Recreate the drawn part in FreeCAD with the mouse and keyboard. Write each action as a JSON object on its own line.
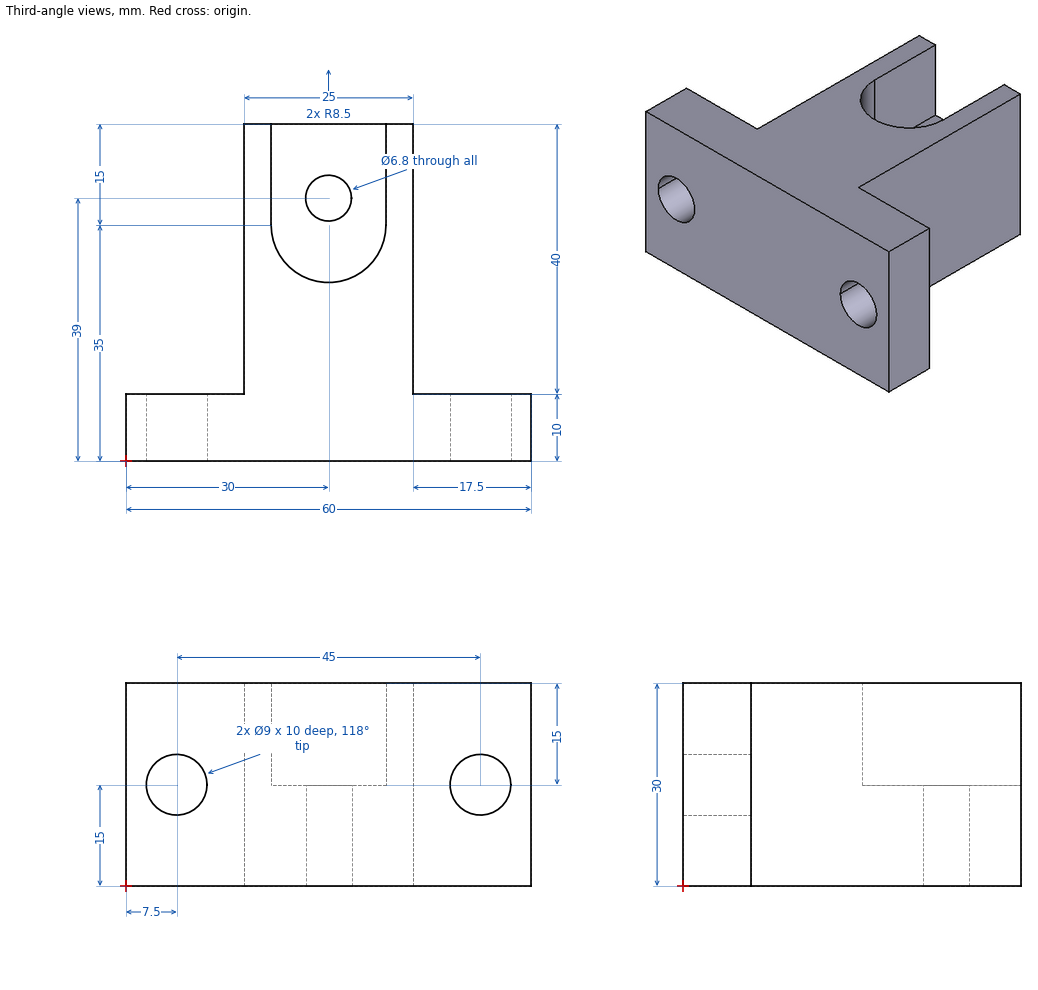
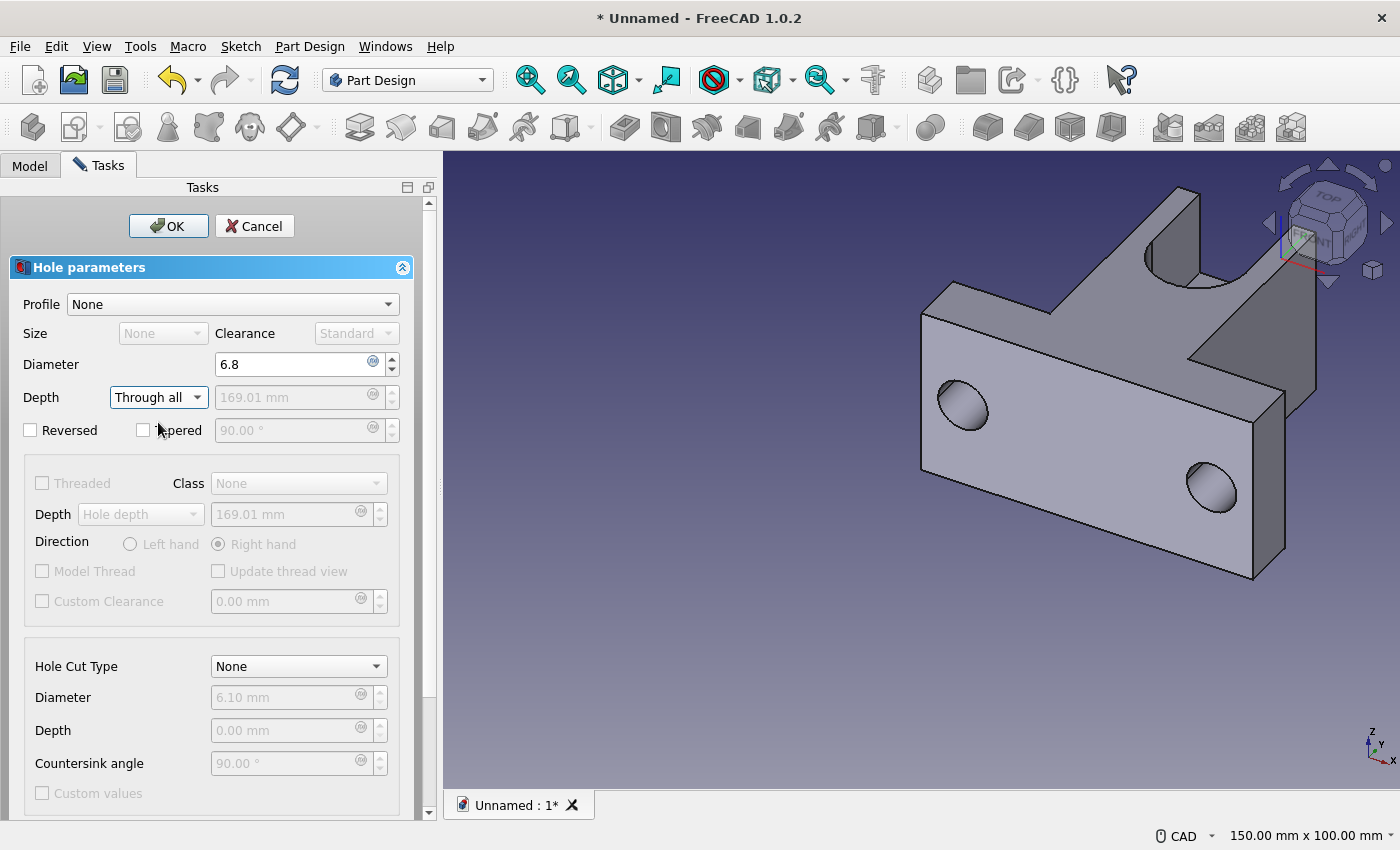
{"action": "left_click", "coordinate": [31, 430]}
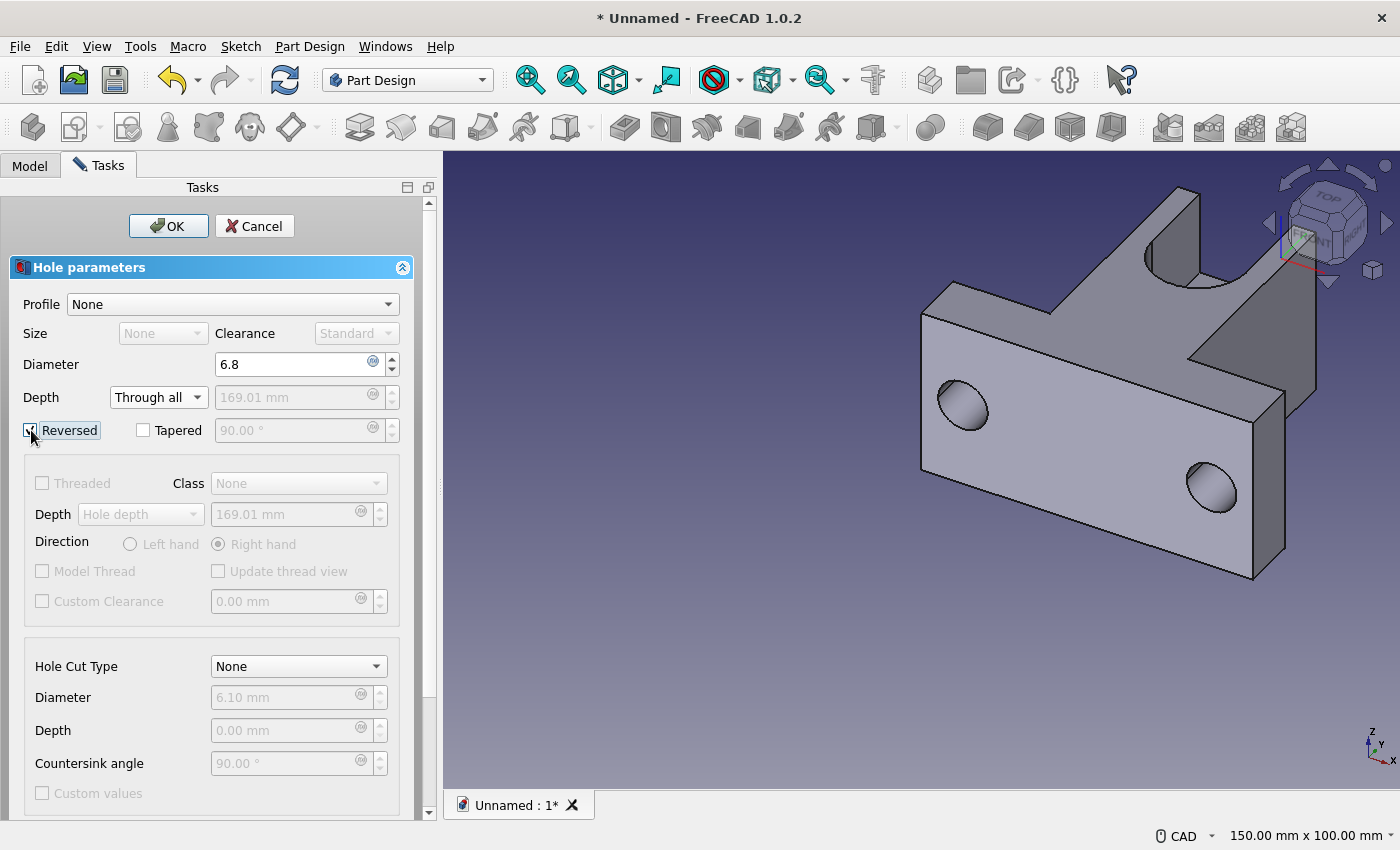
{"action": "left_click", "coordinate": [169, 226]}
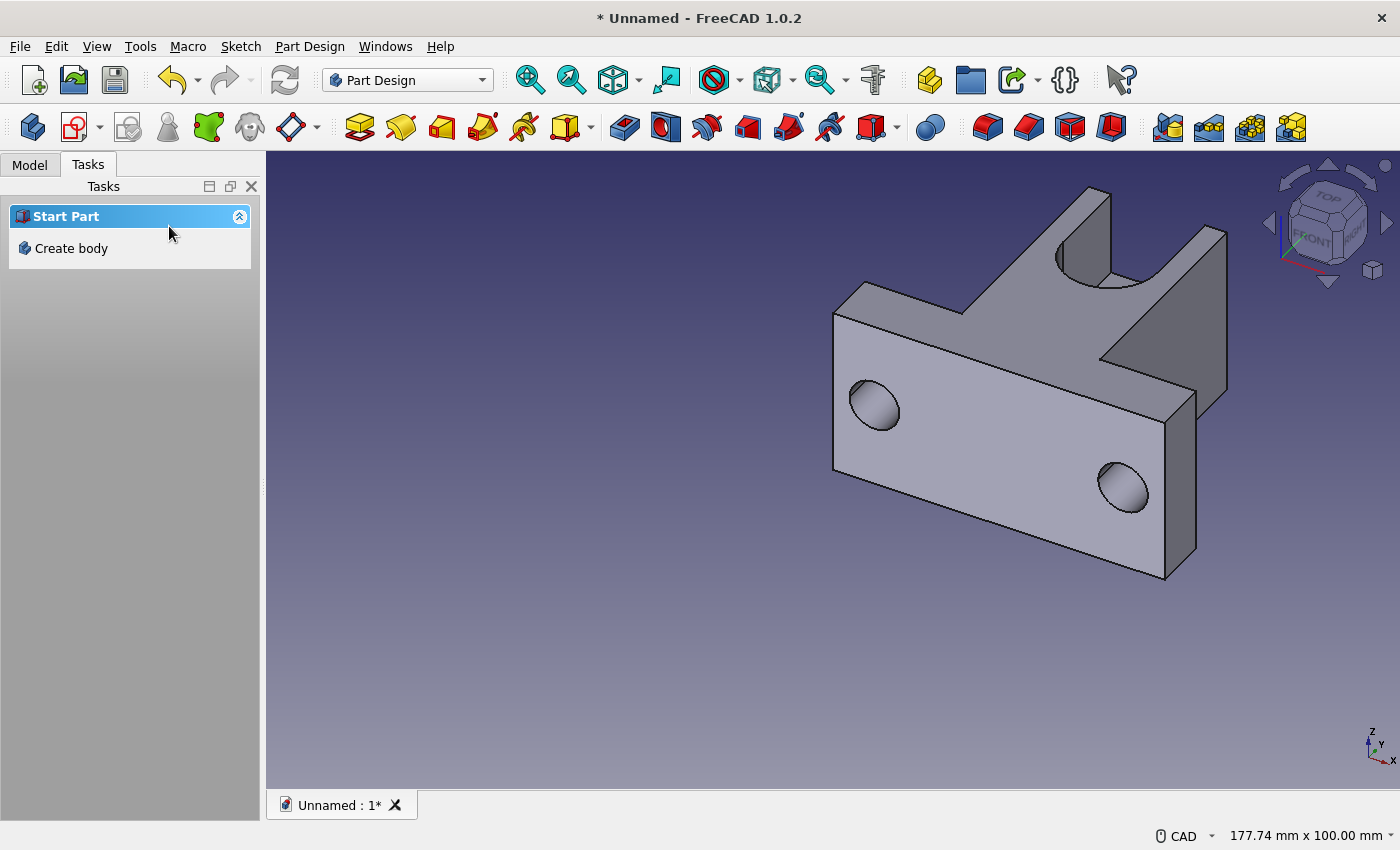
{"action": "key", "text": "0"}